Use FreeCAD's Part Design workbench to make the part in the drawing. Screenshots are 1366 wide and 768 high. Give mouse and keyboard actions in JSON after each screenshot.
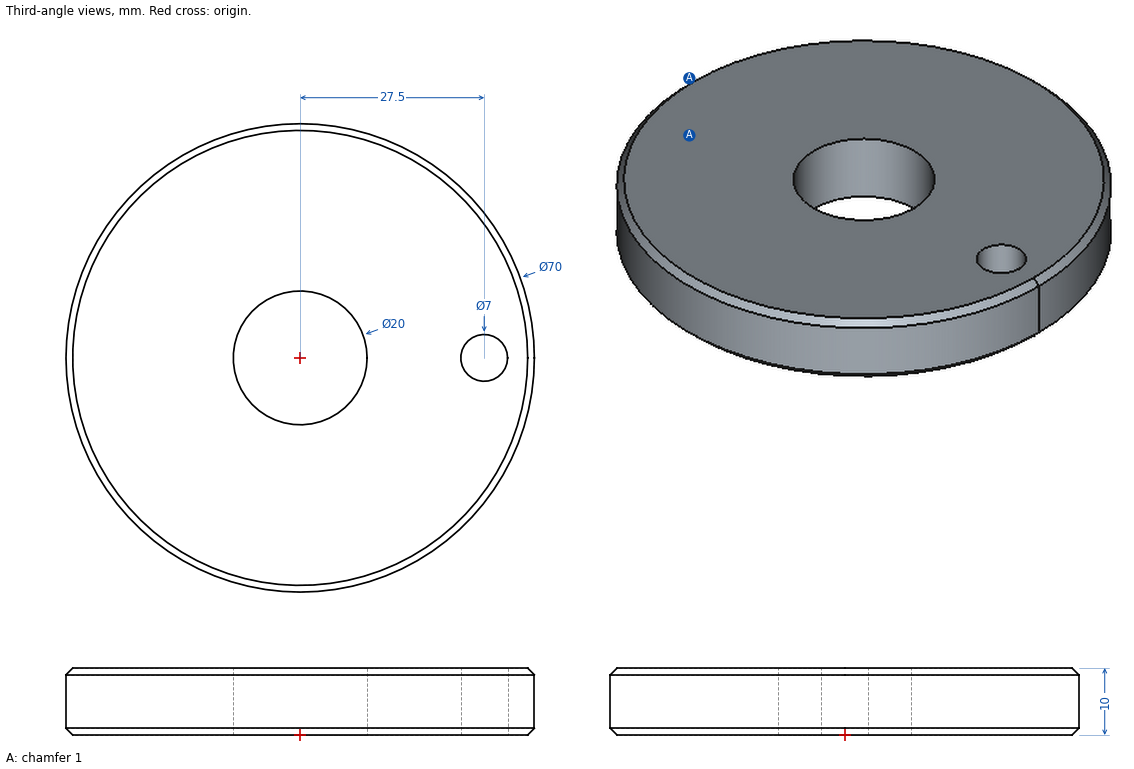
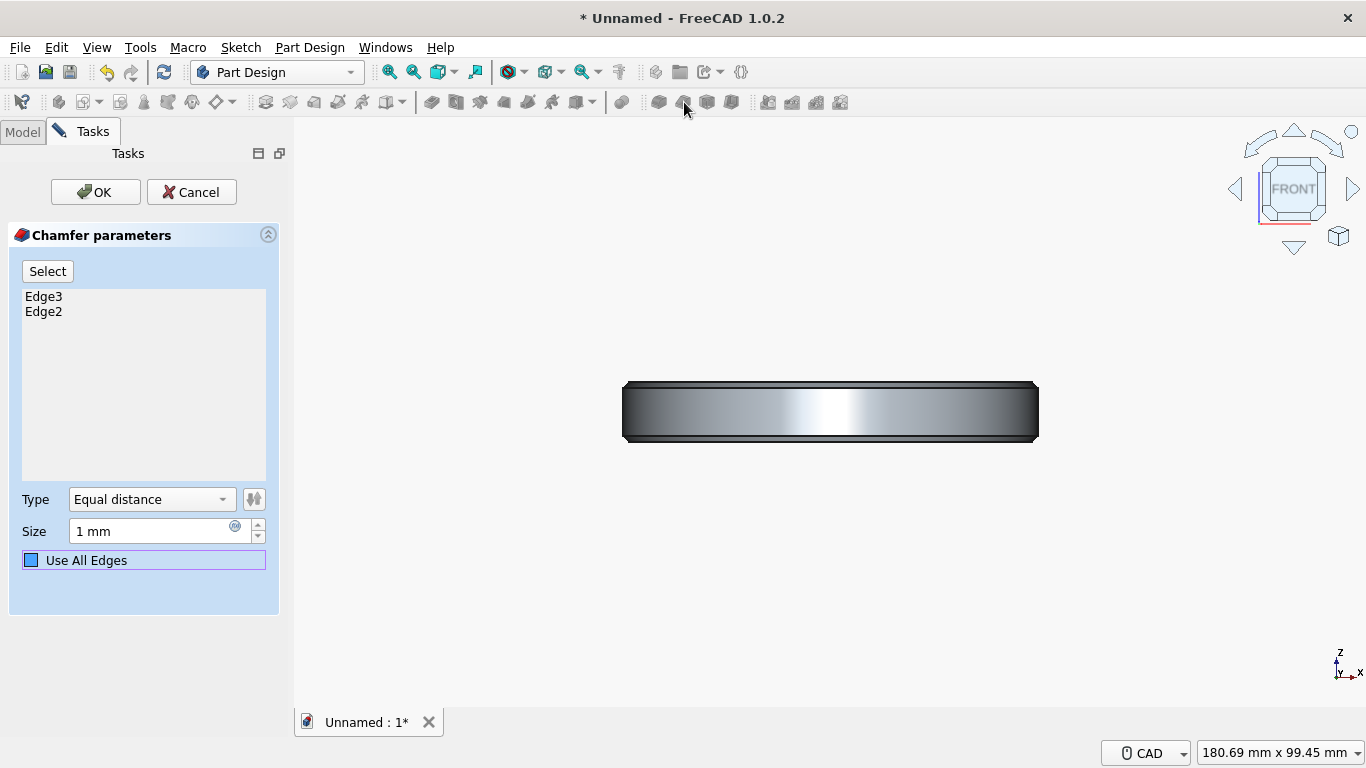
{"action": "left_click", "coordinate": [96, 192]}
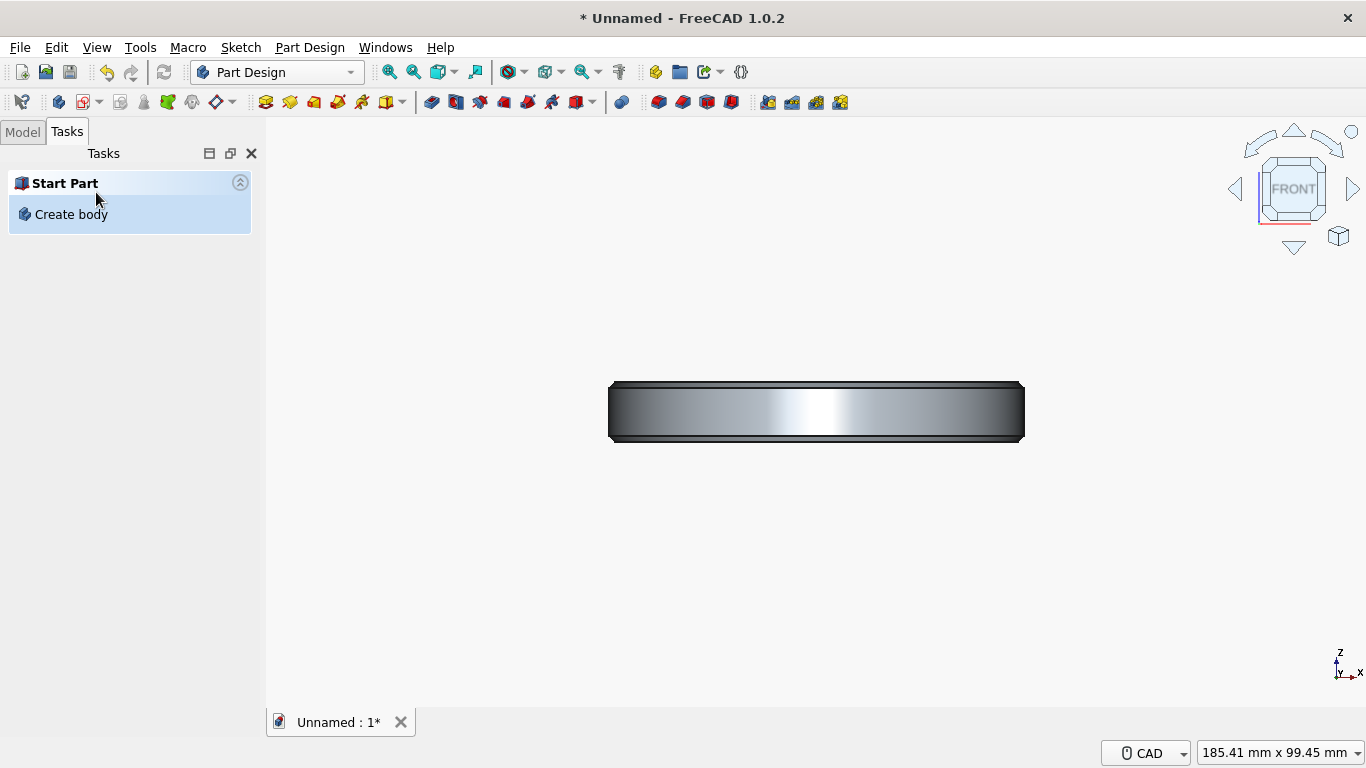
{"action": "left_click", "coordinate": [390, 72]}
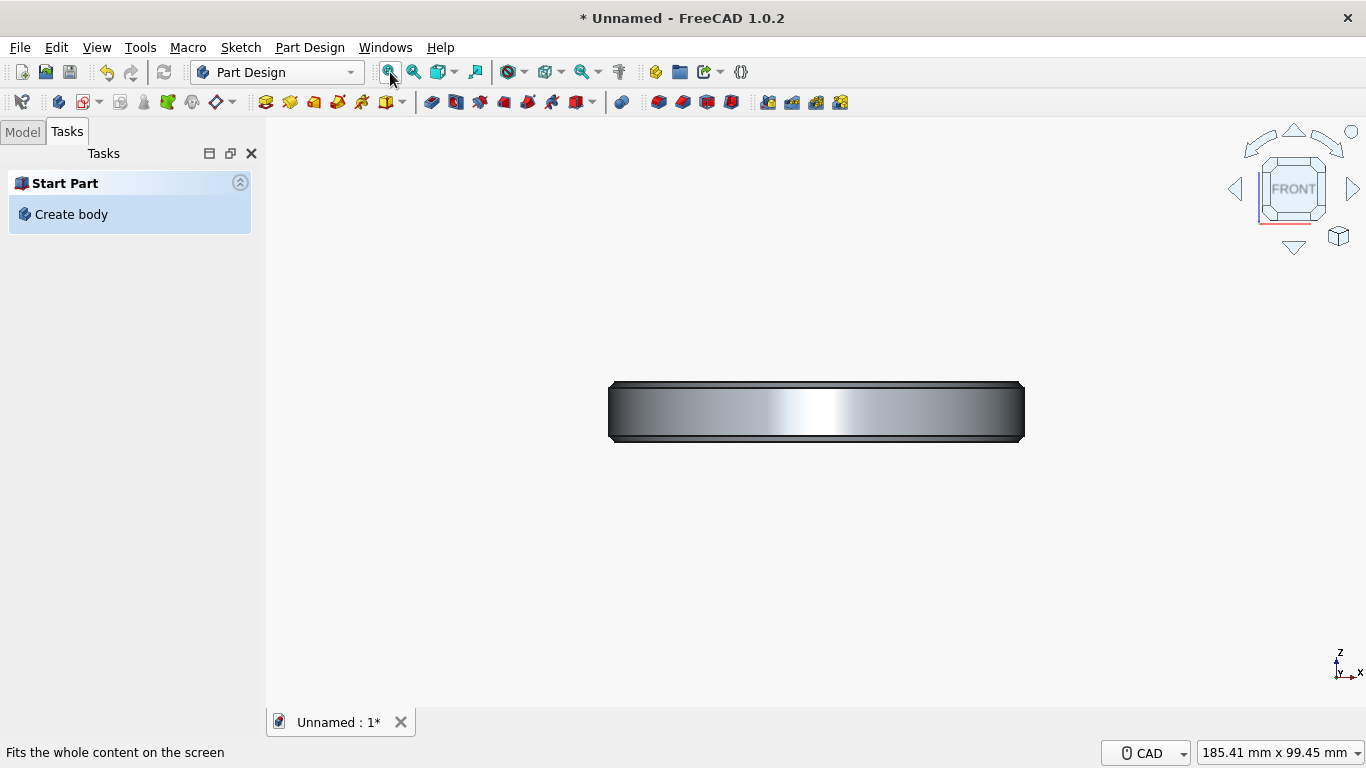
{"action": "key", "text": "0"}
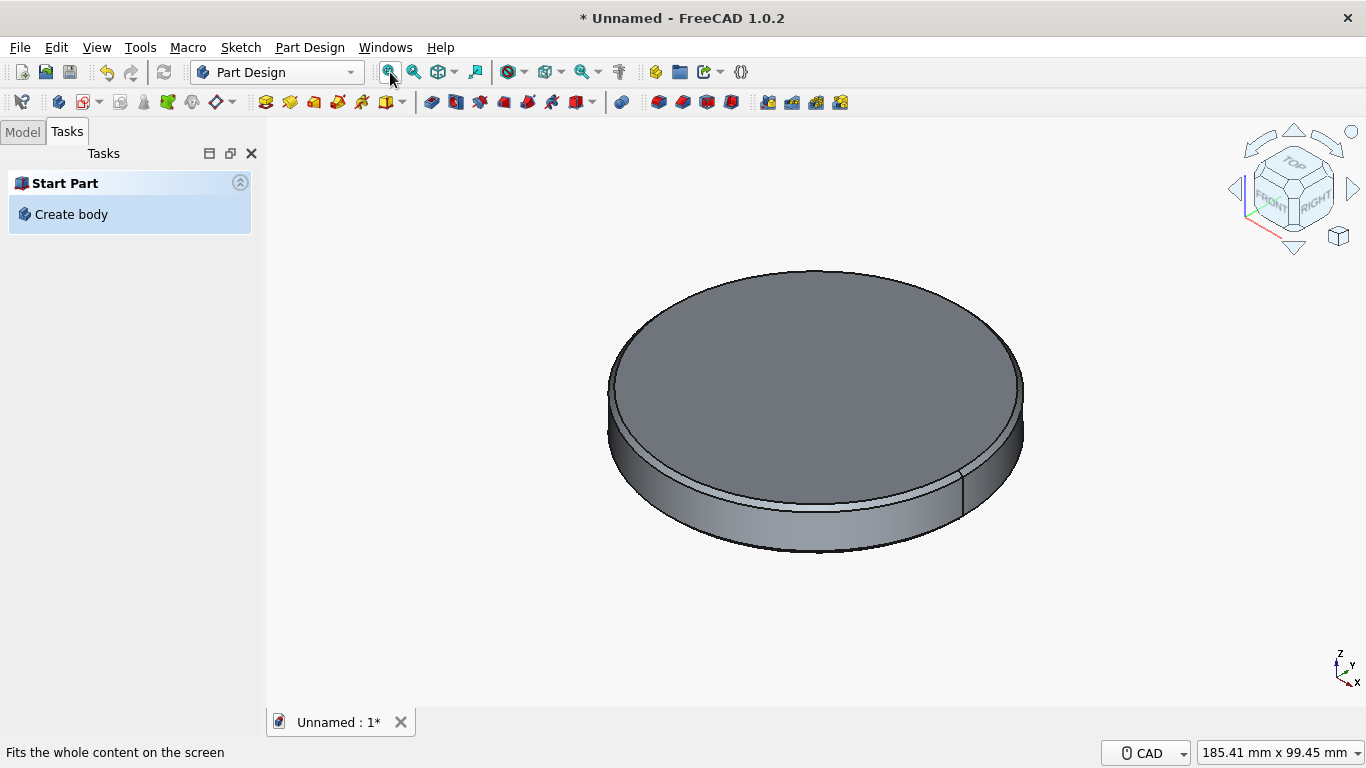
{"action": "left_click", "coordinate": [816, 387]}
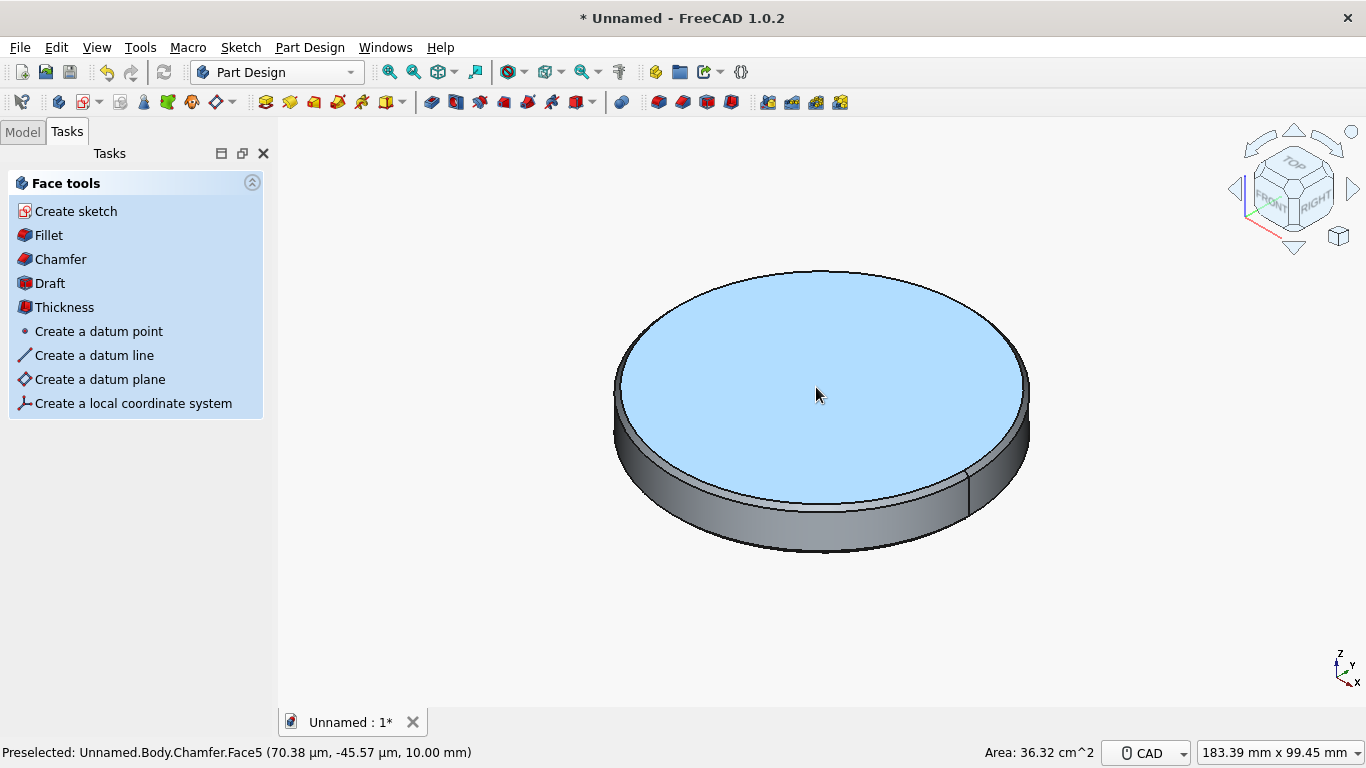
{"action": "left_click", "coordinate": [84, 102]}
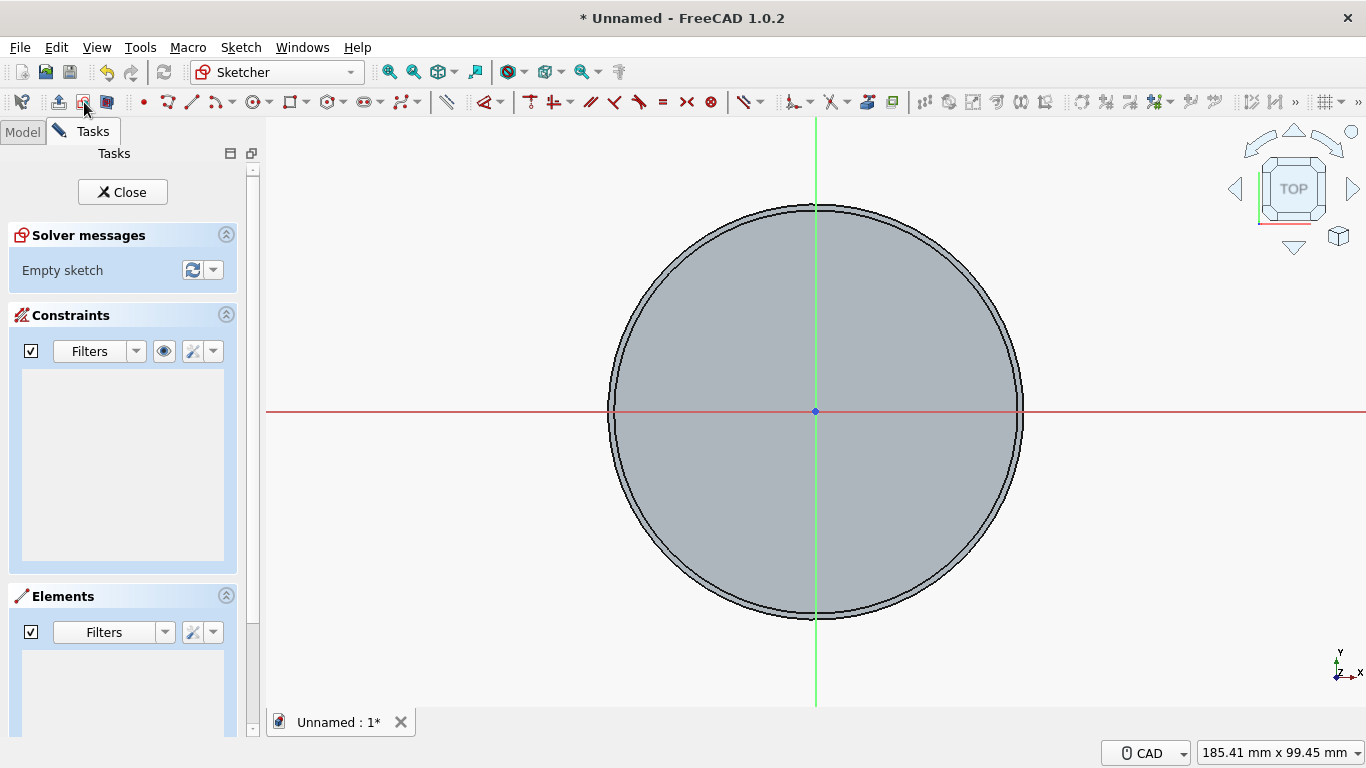
{"action": "scroll", "coordinate": [845, 412], "scroll_direction": "up", "scroll_amount": 6}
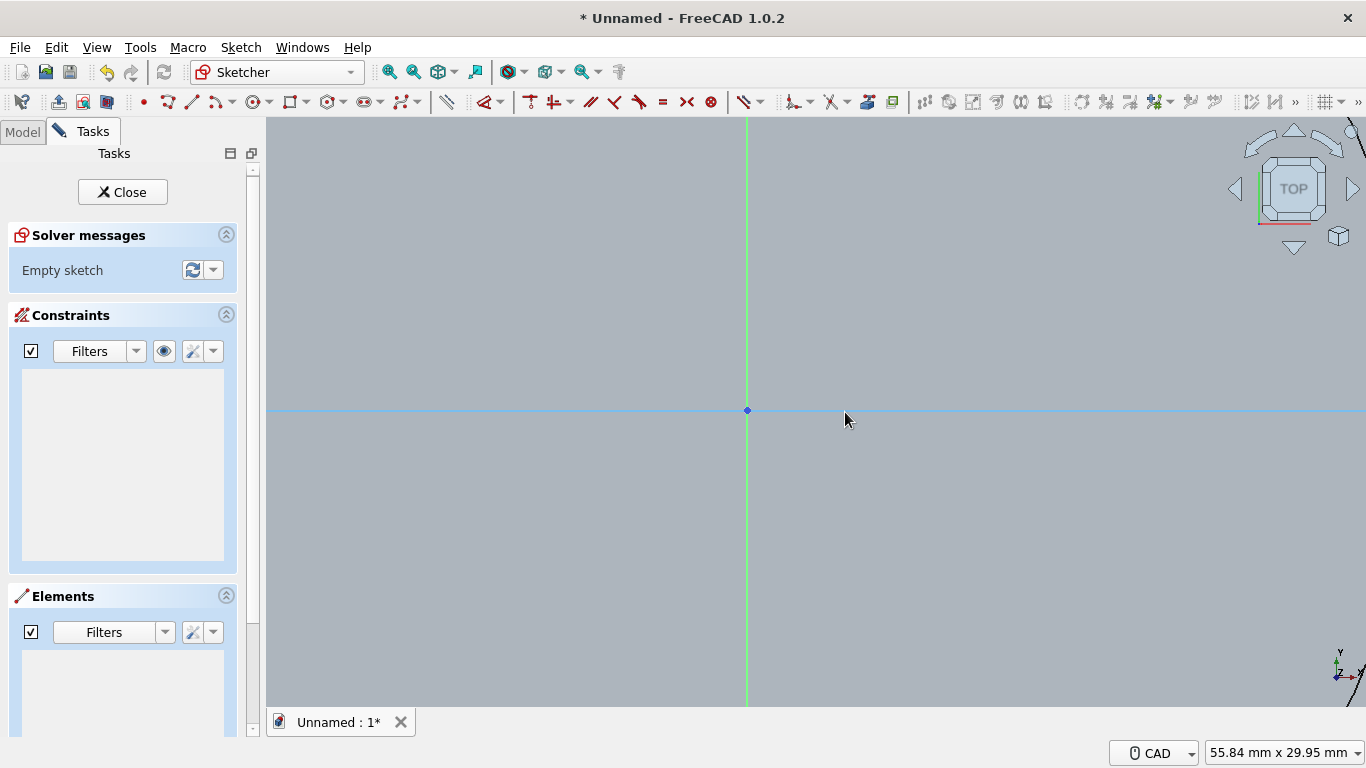
{"action": "left_click", "coordinate": [254, 102]}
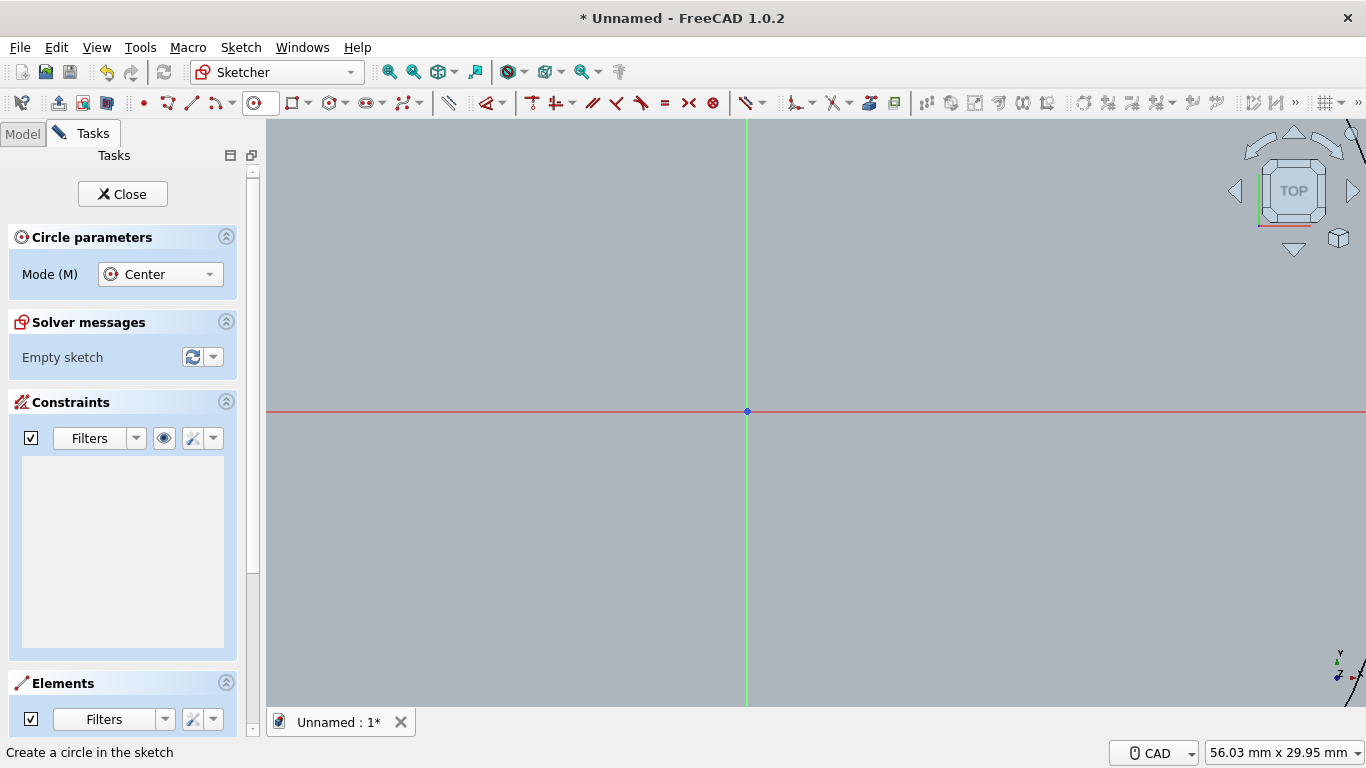
{"action": "left_click", "coordinate": [747, 412]}
{"action": "mouse_move", "coordinate": [886, 273]}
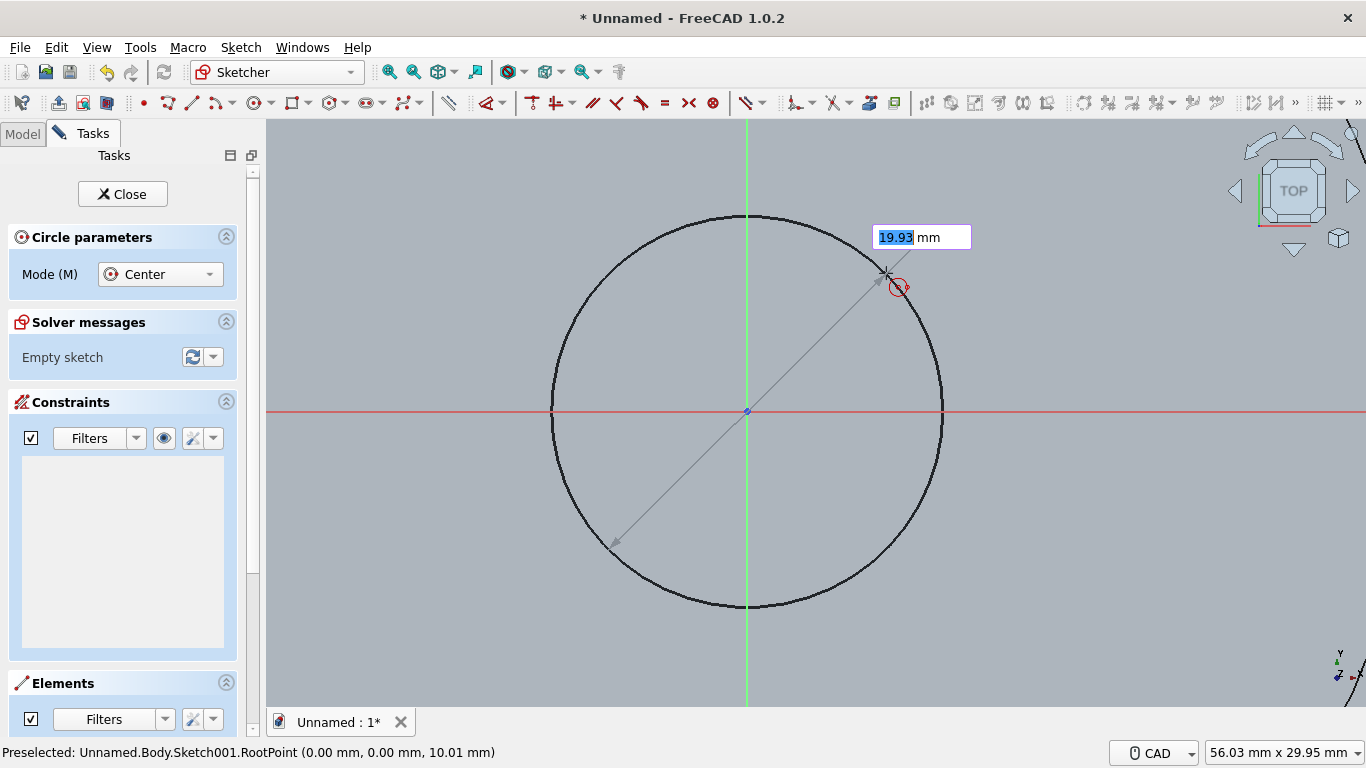
{"action": "type", "text": "20"}
{"action": "key", "text": "Return"}
{"action": "key", "text": "Escape"}